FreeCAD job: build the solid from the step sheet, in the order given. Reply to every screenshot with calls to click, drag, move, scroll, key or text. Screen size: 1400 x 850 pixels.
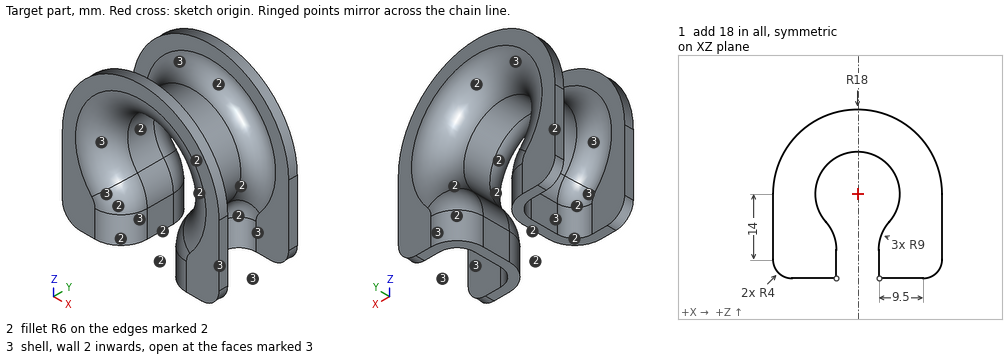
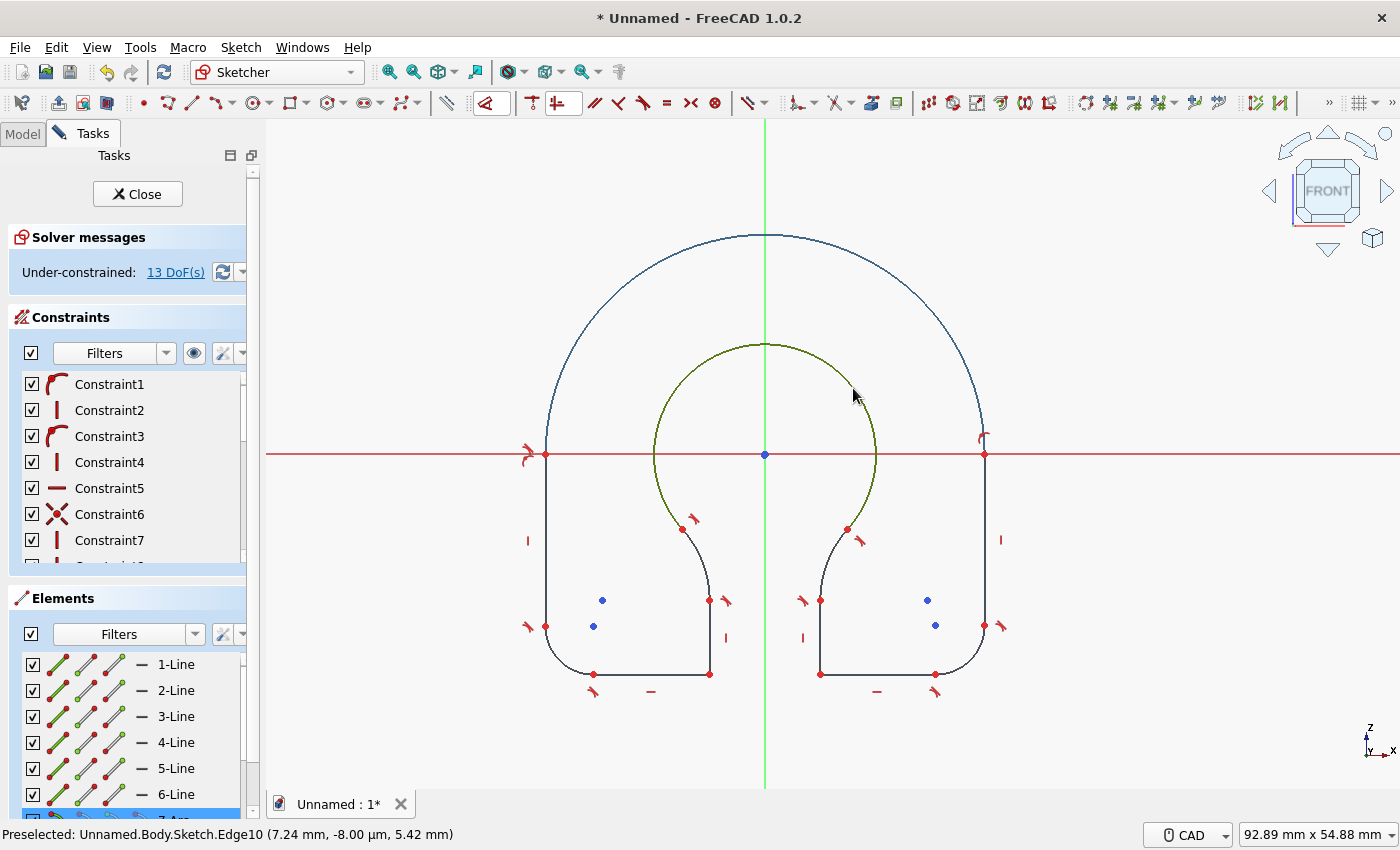
click(532, 104)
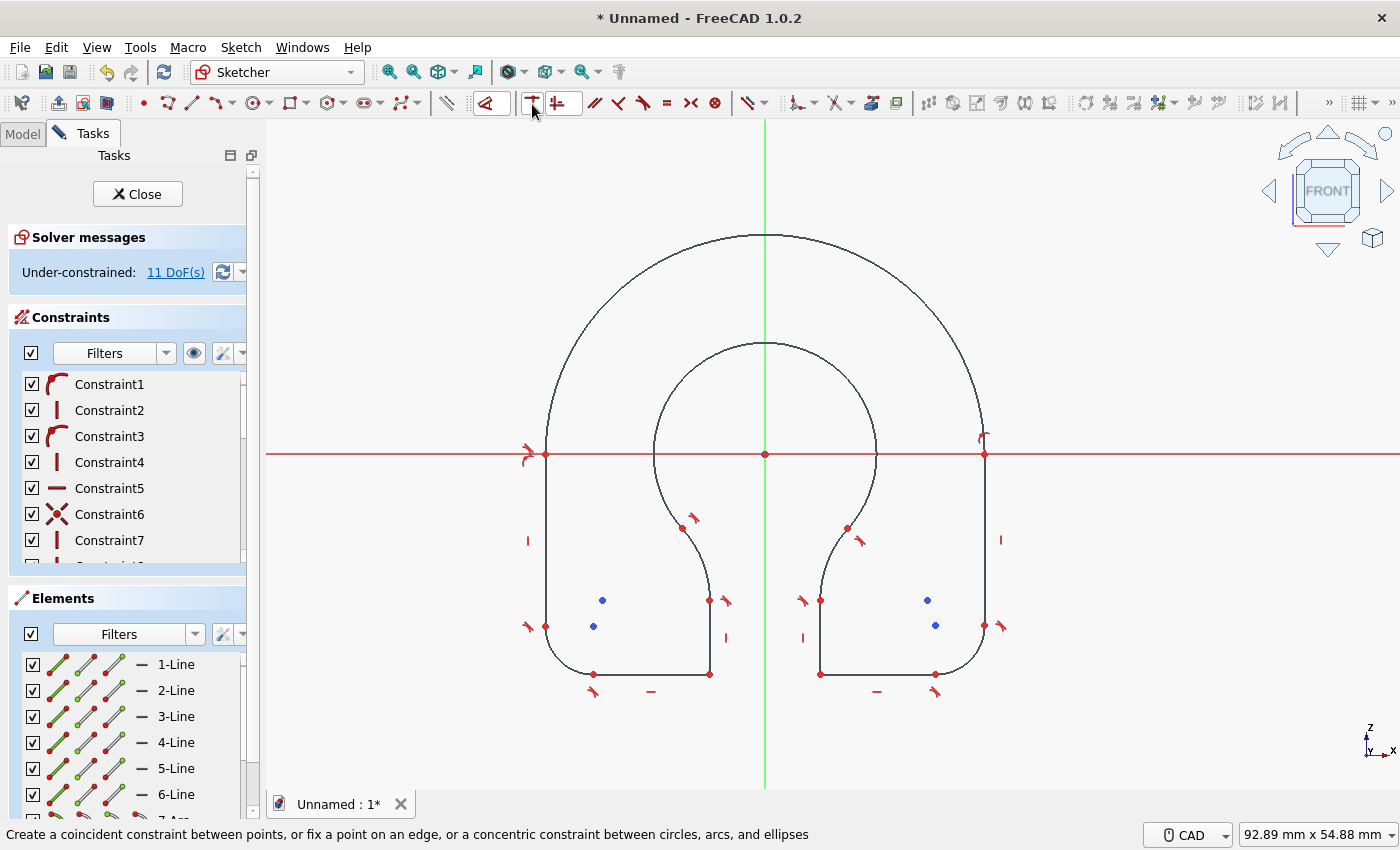
click(834, 548)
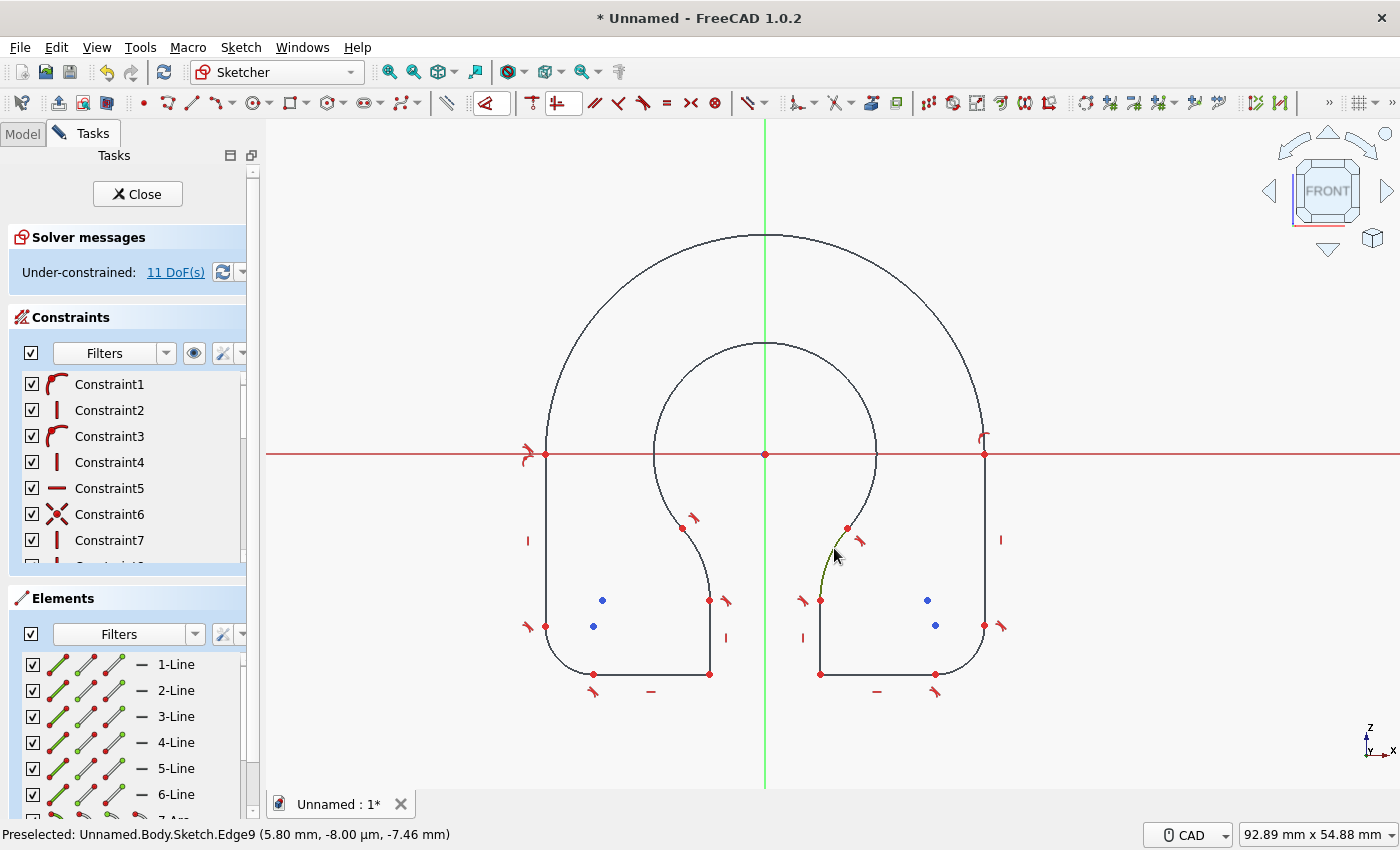
click(854, 387)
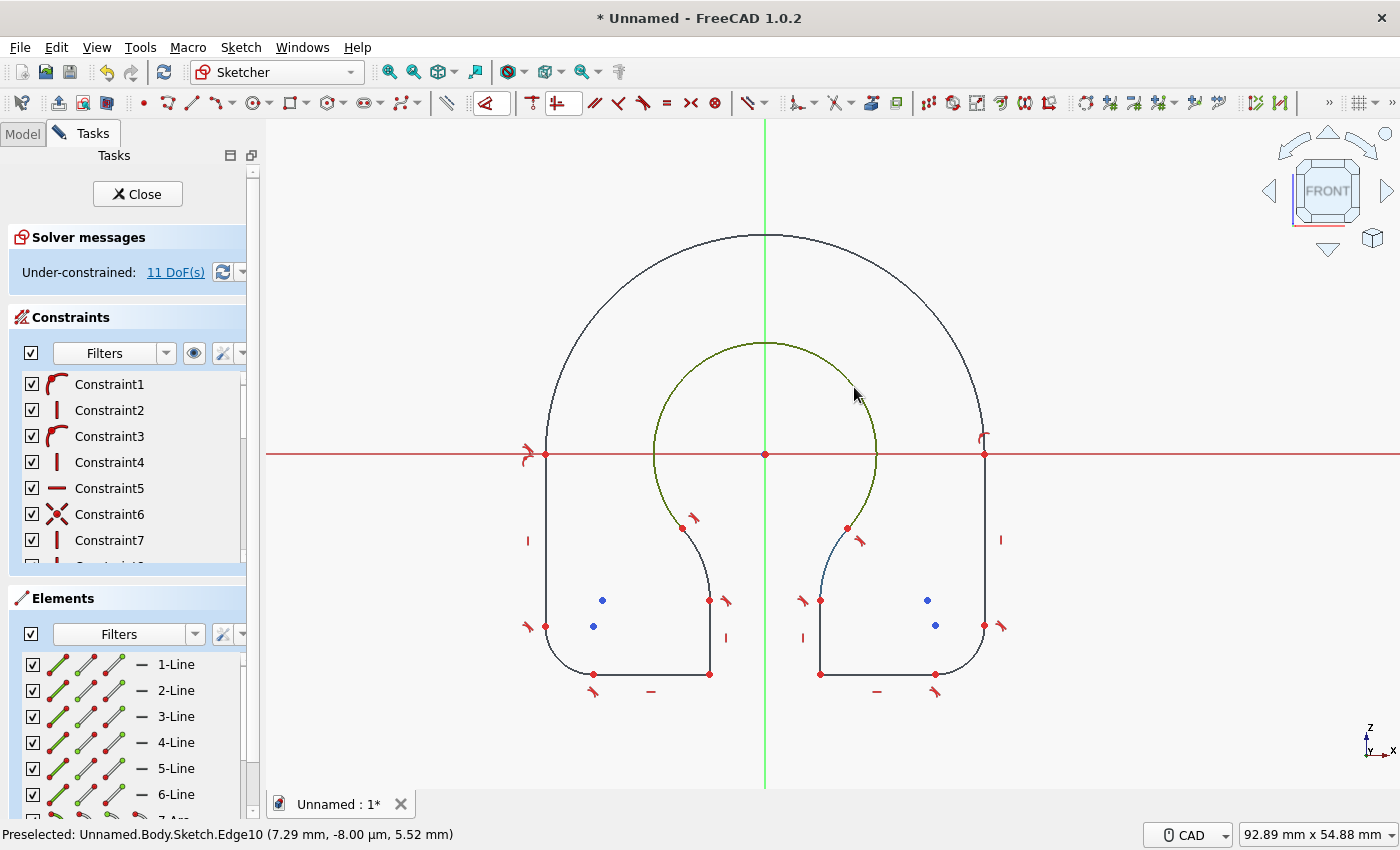
click(707, 577)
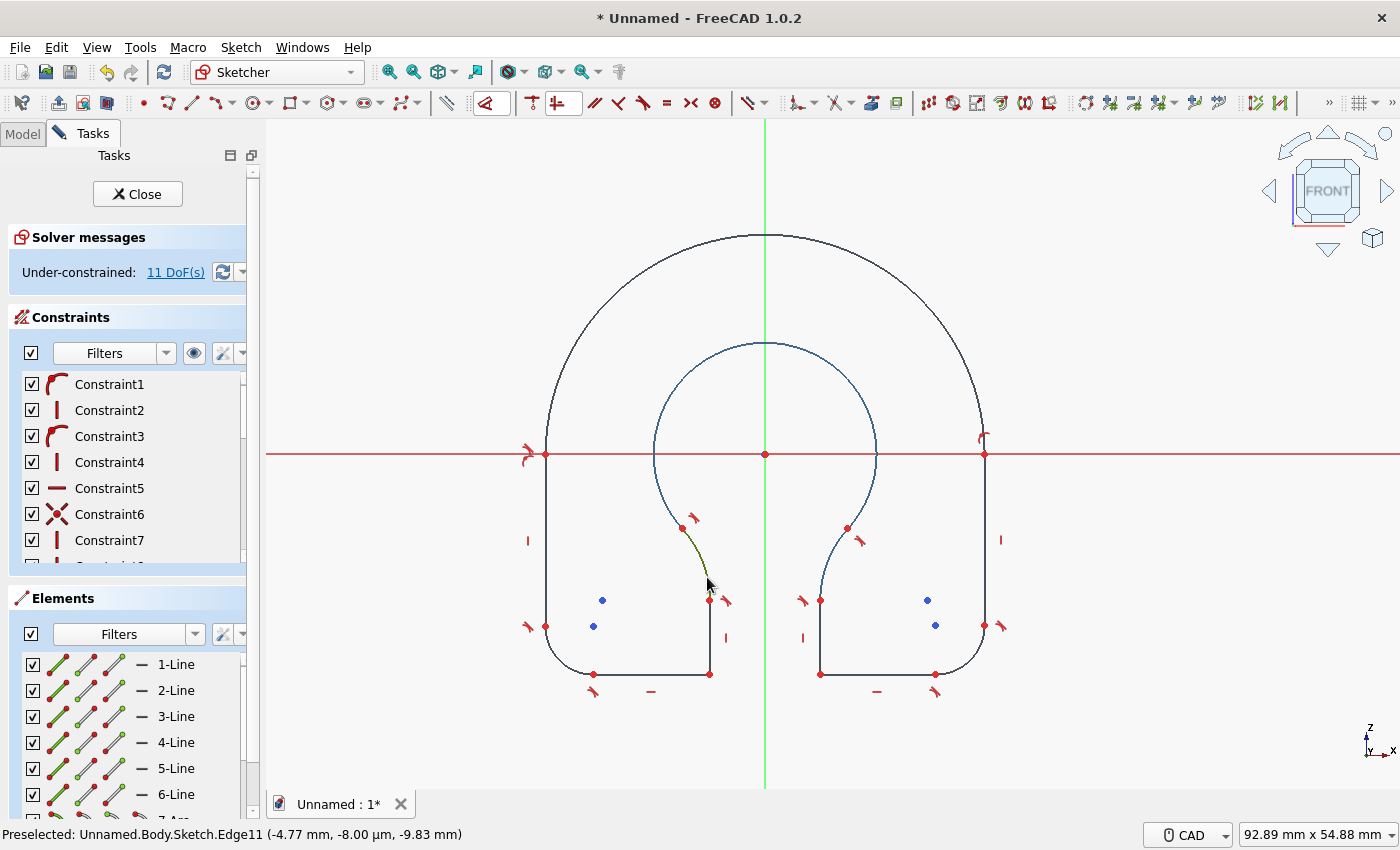
key(e)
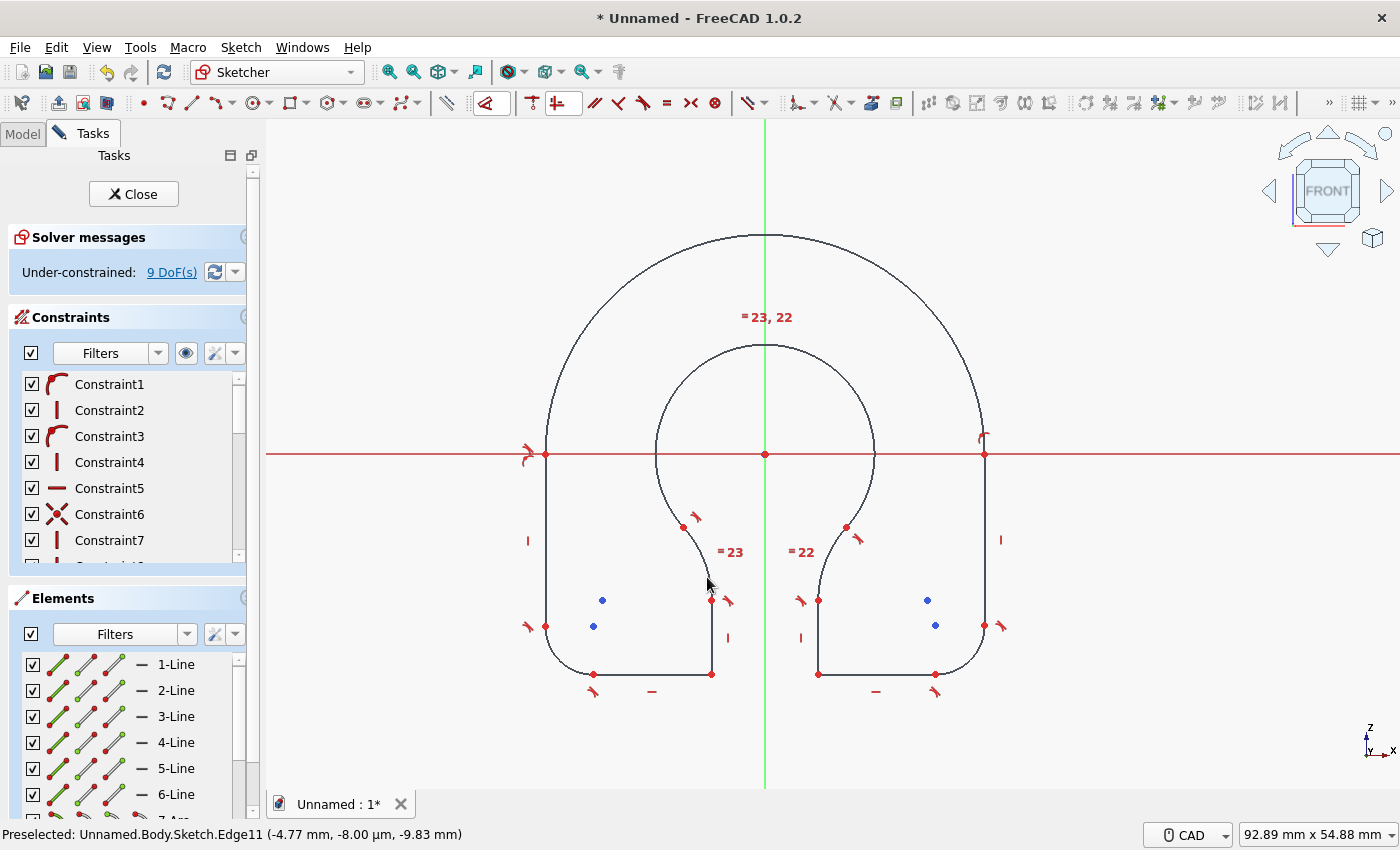
click(958, 669)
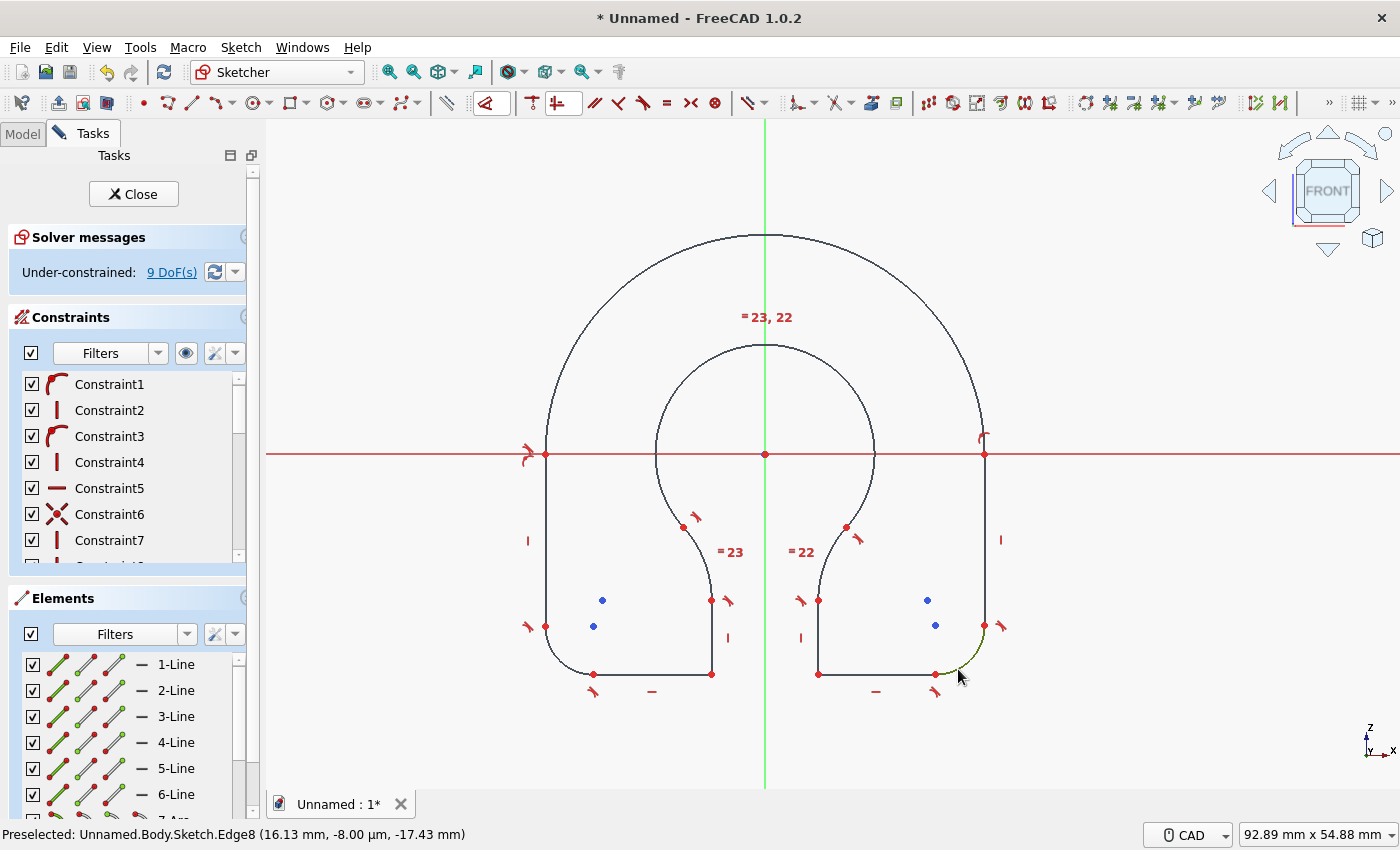
click(551, 648)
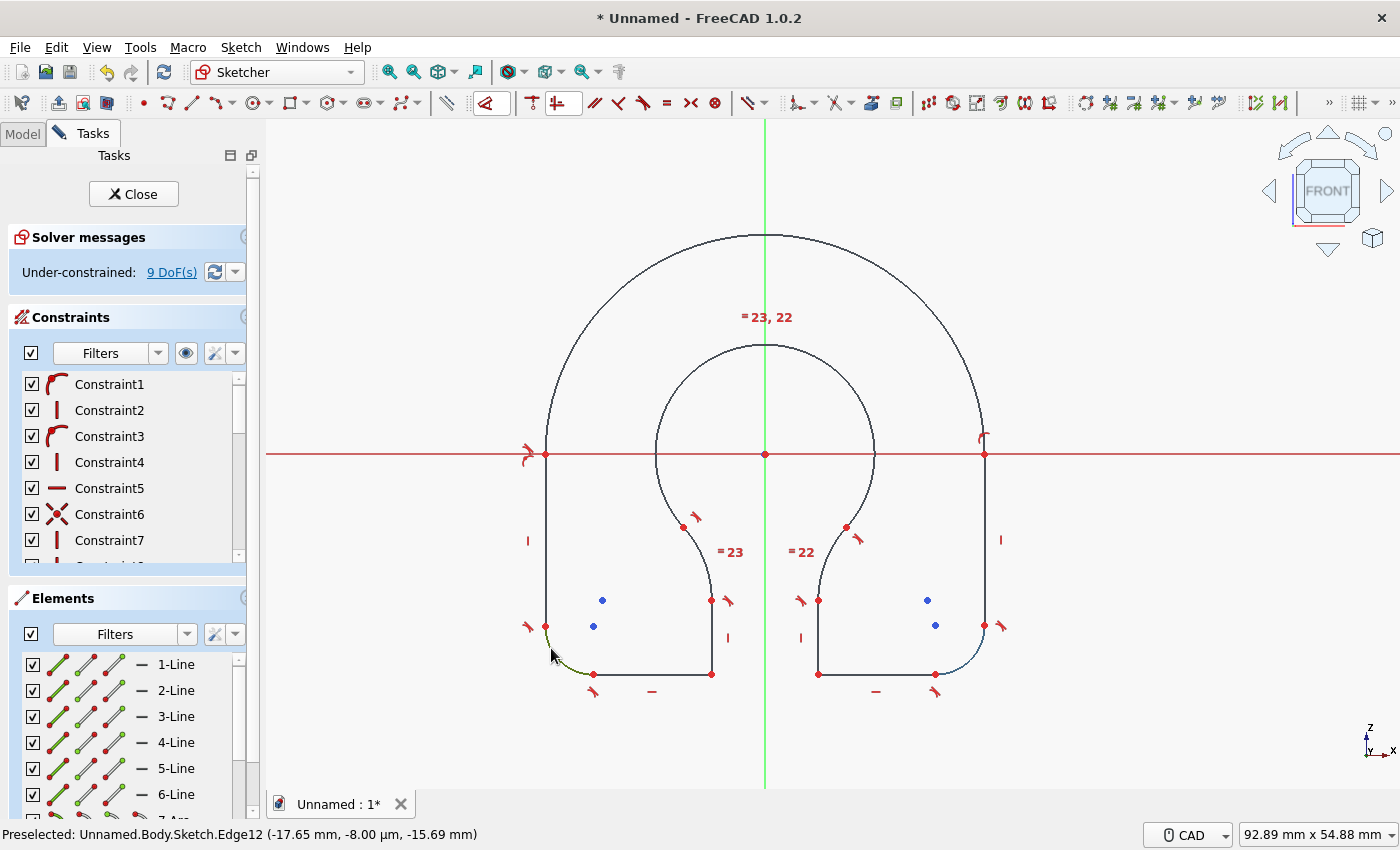
key(e)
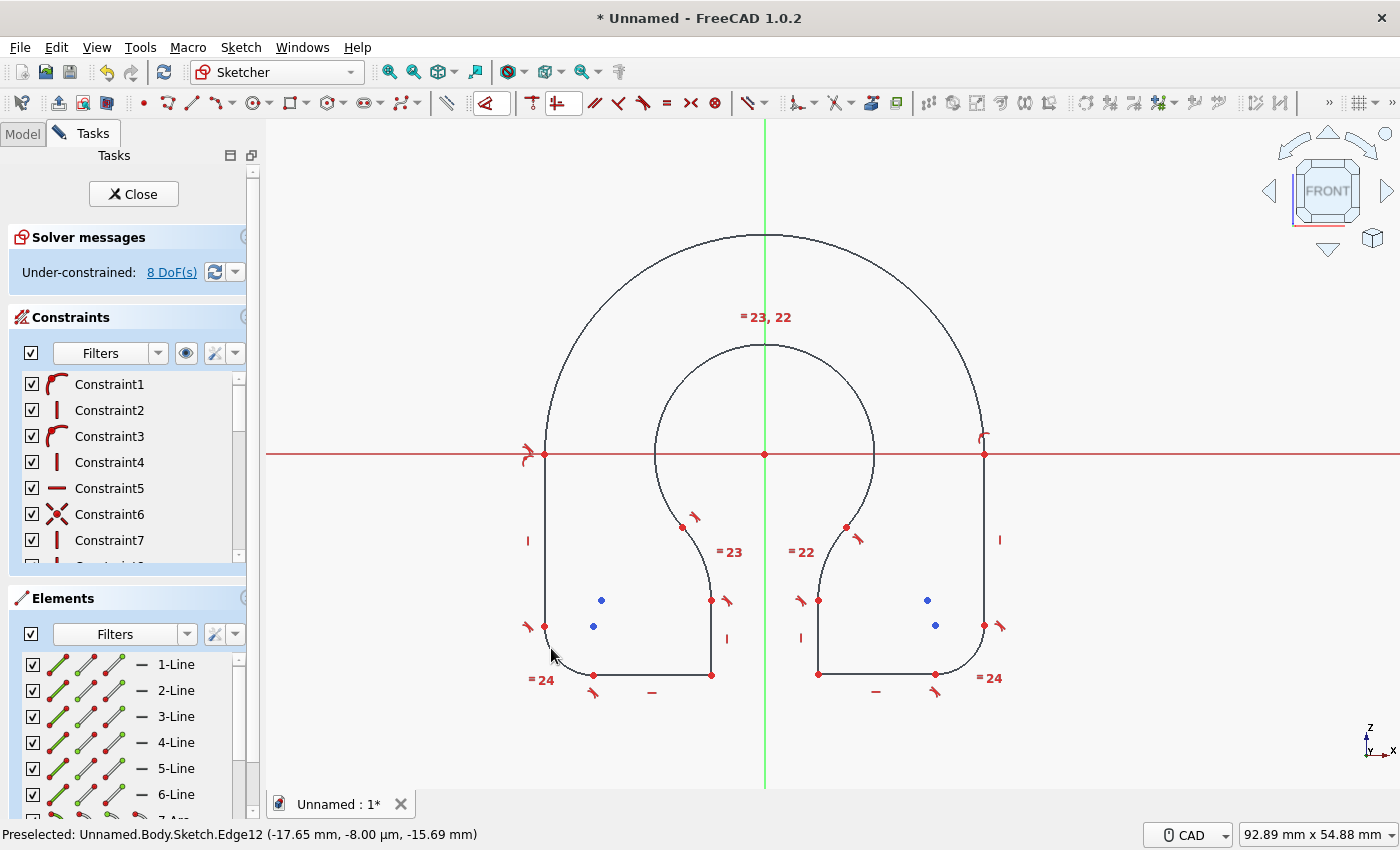
click(765, 454)